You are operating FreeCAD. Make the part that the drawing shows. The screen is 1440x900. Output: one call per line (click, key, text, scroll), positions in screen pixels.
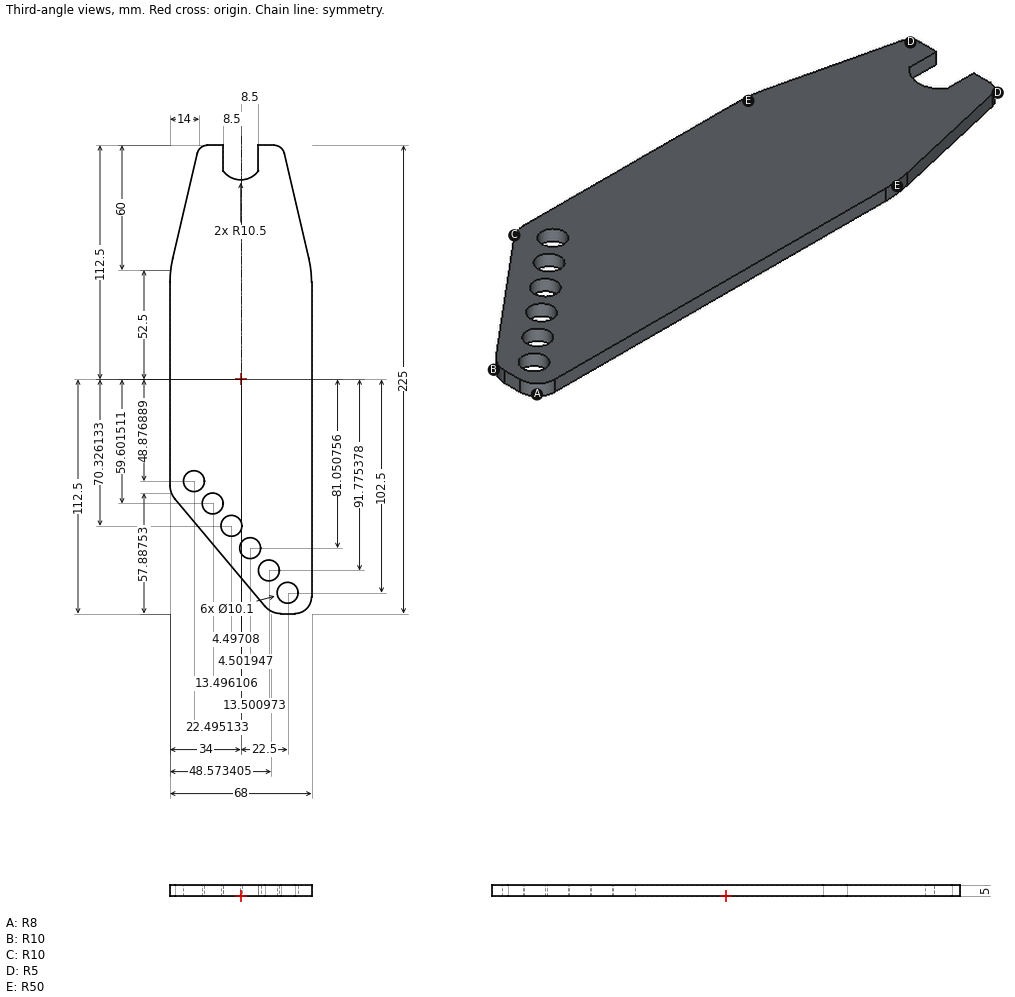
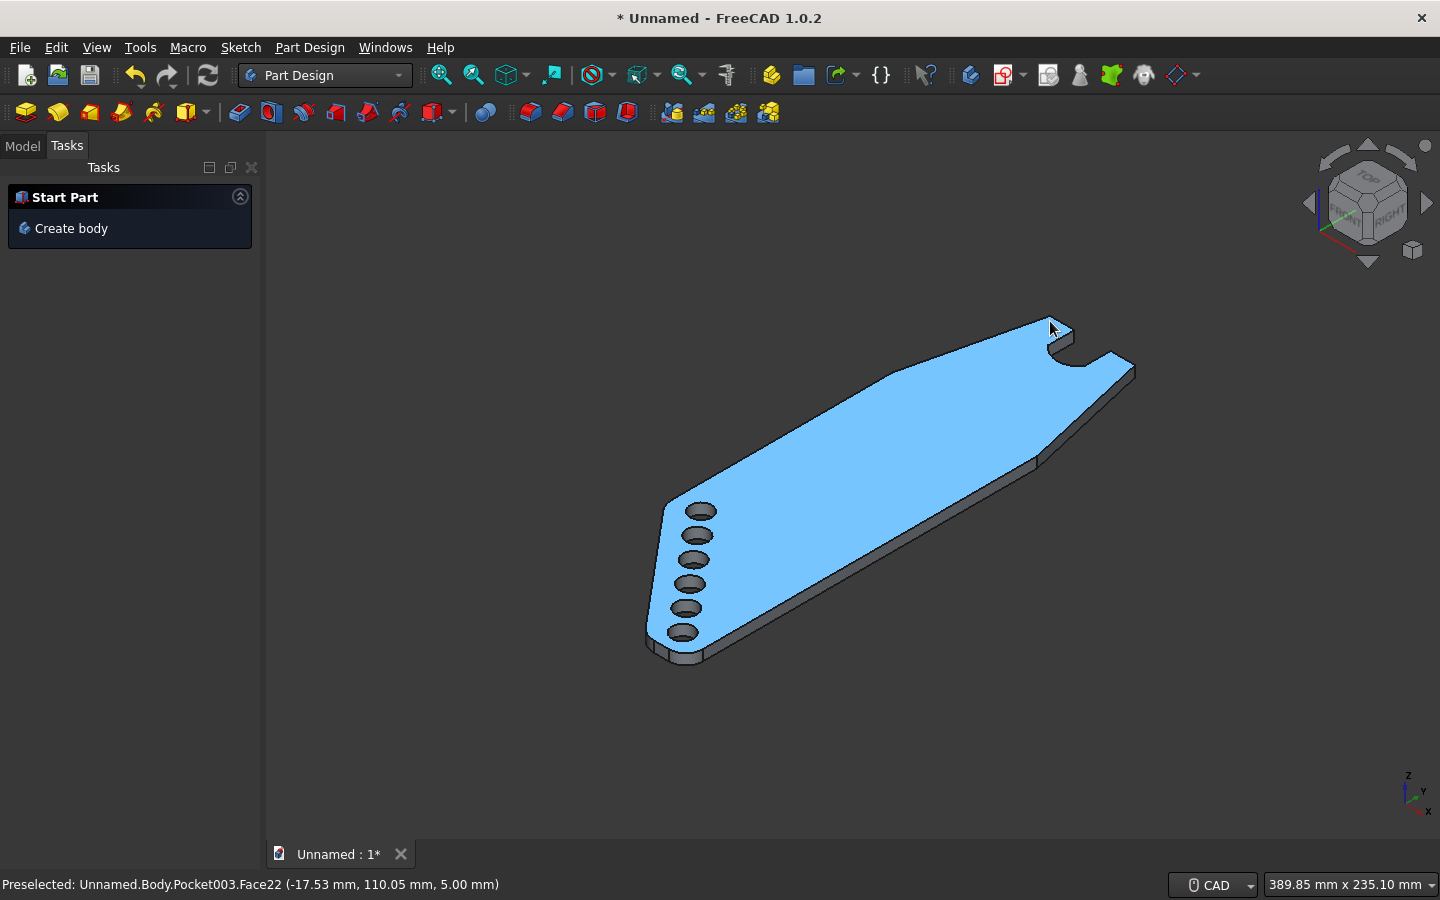
key(2)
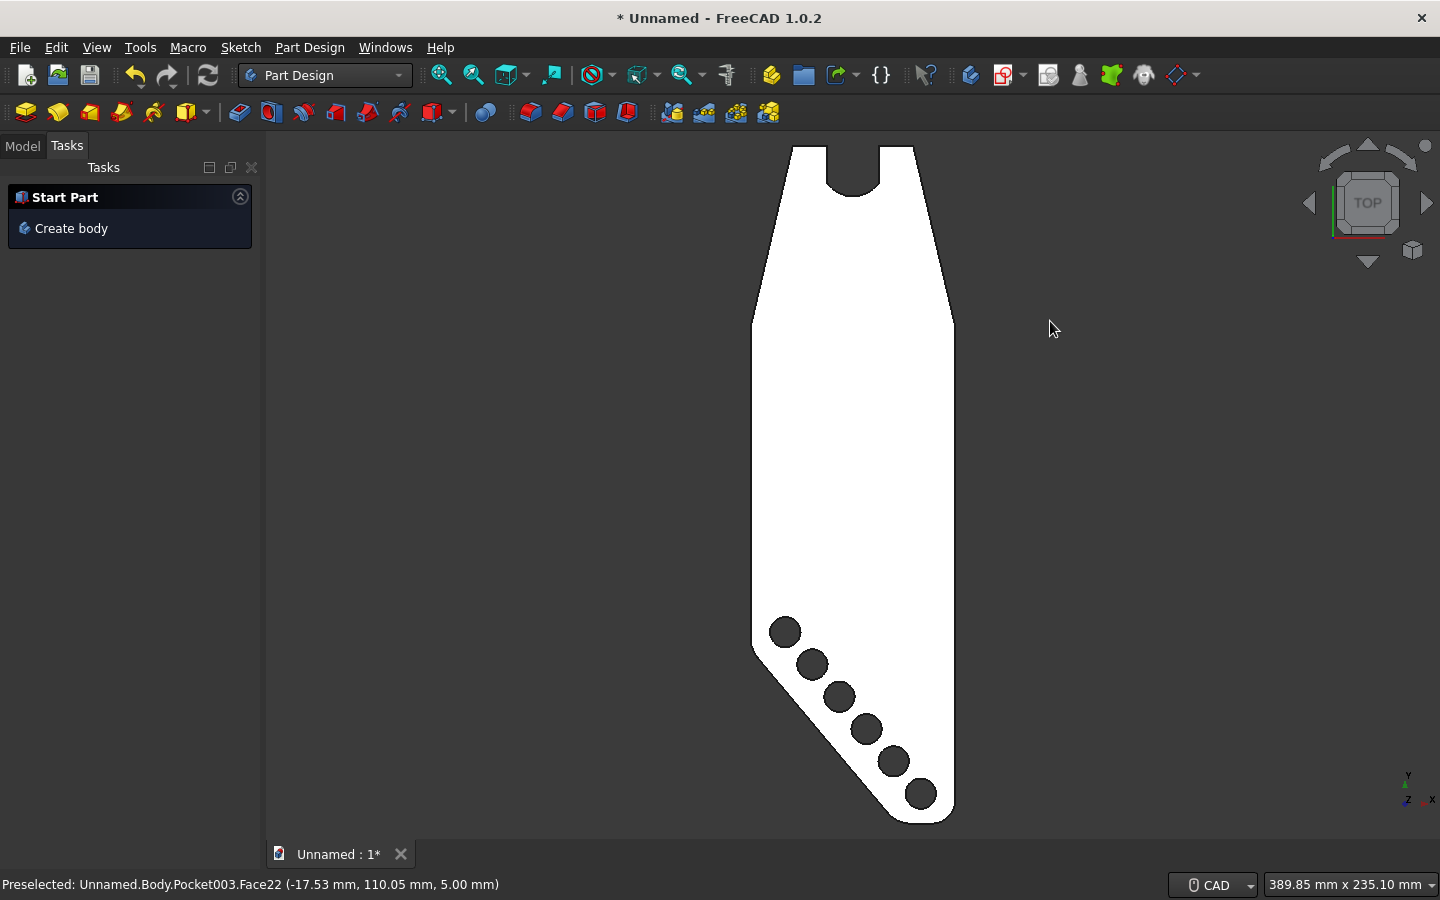
key(0)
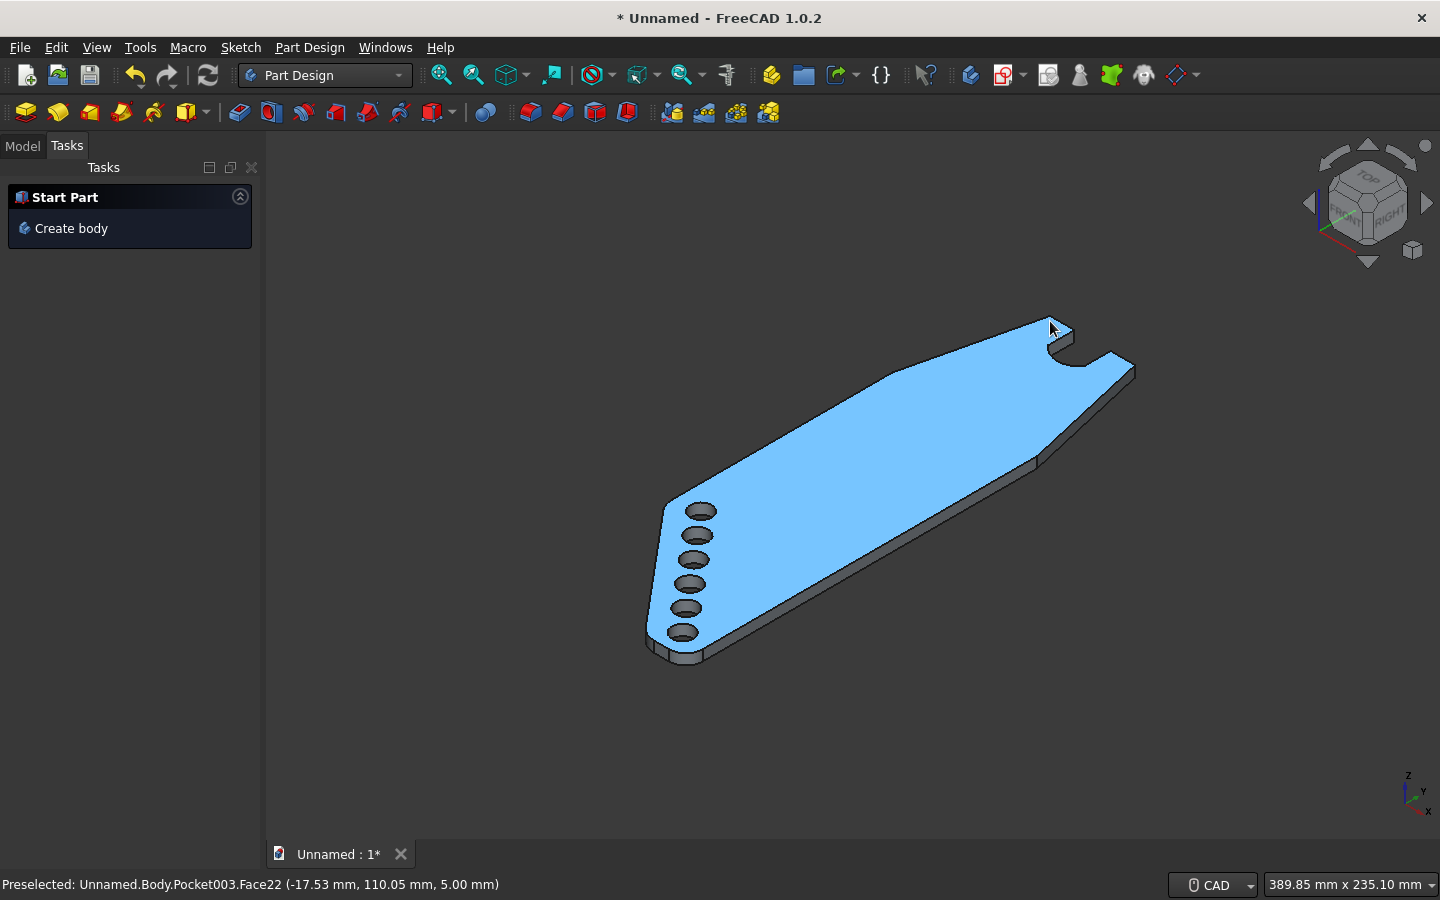
scroll(1050, 321, up, 5)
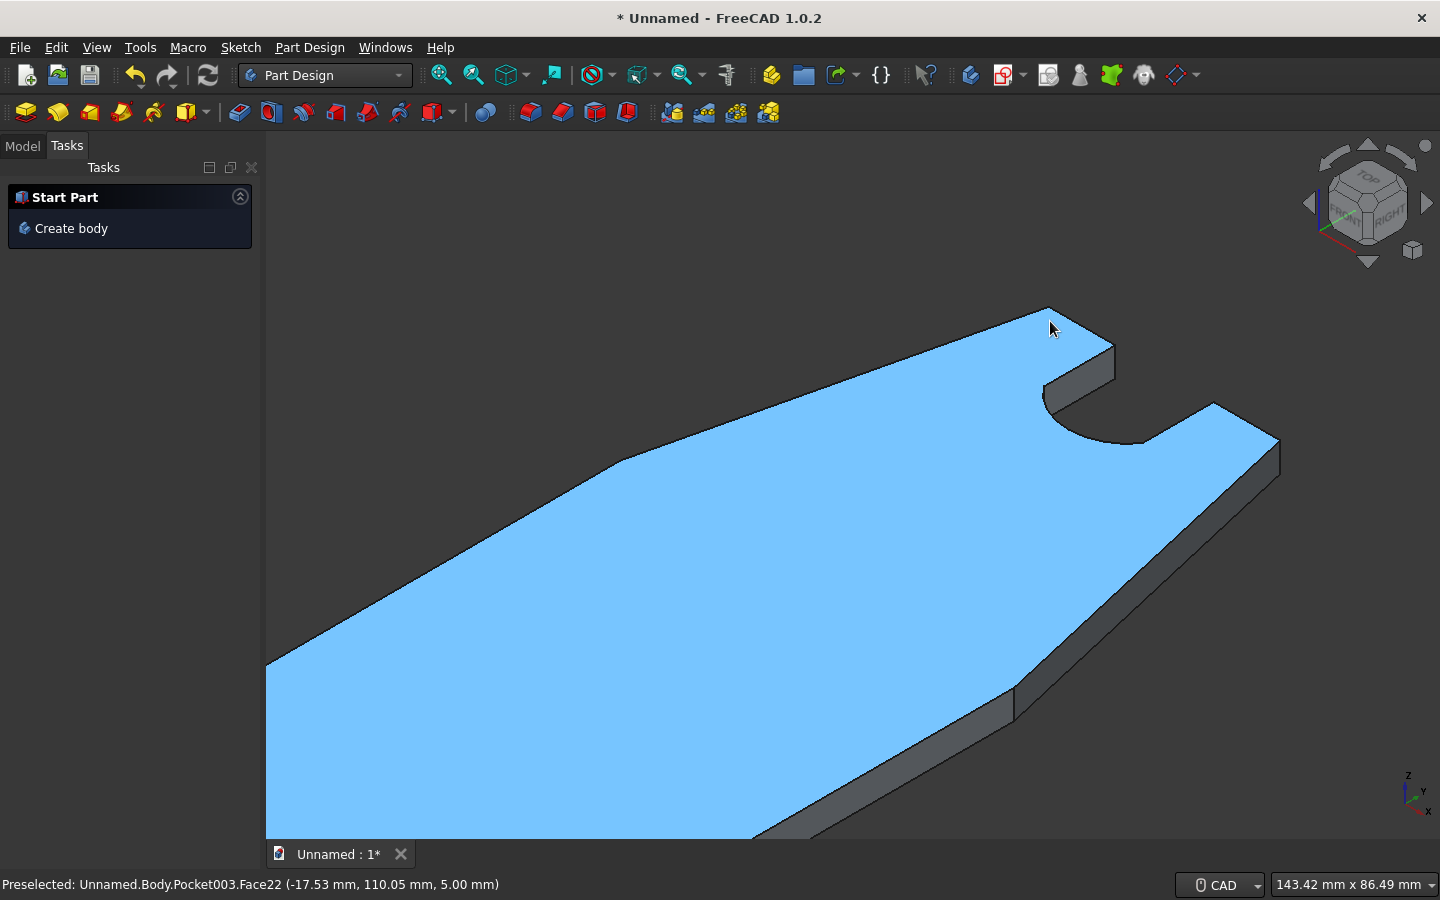
key(v)
key(f)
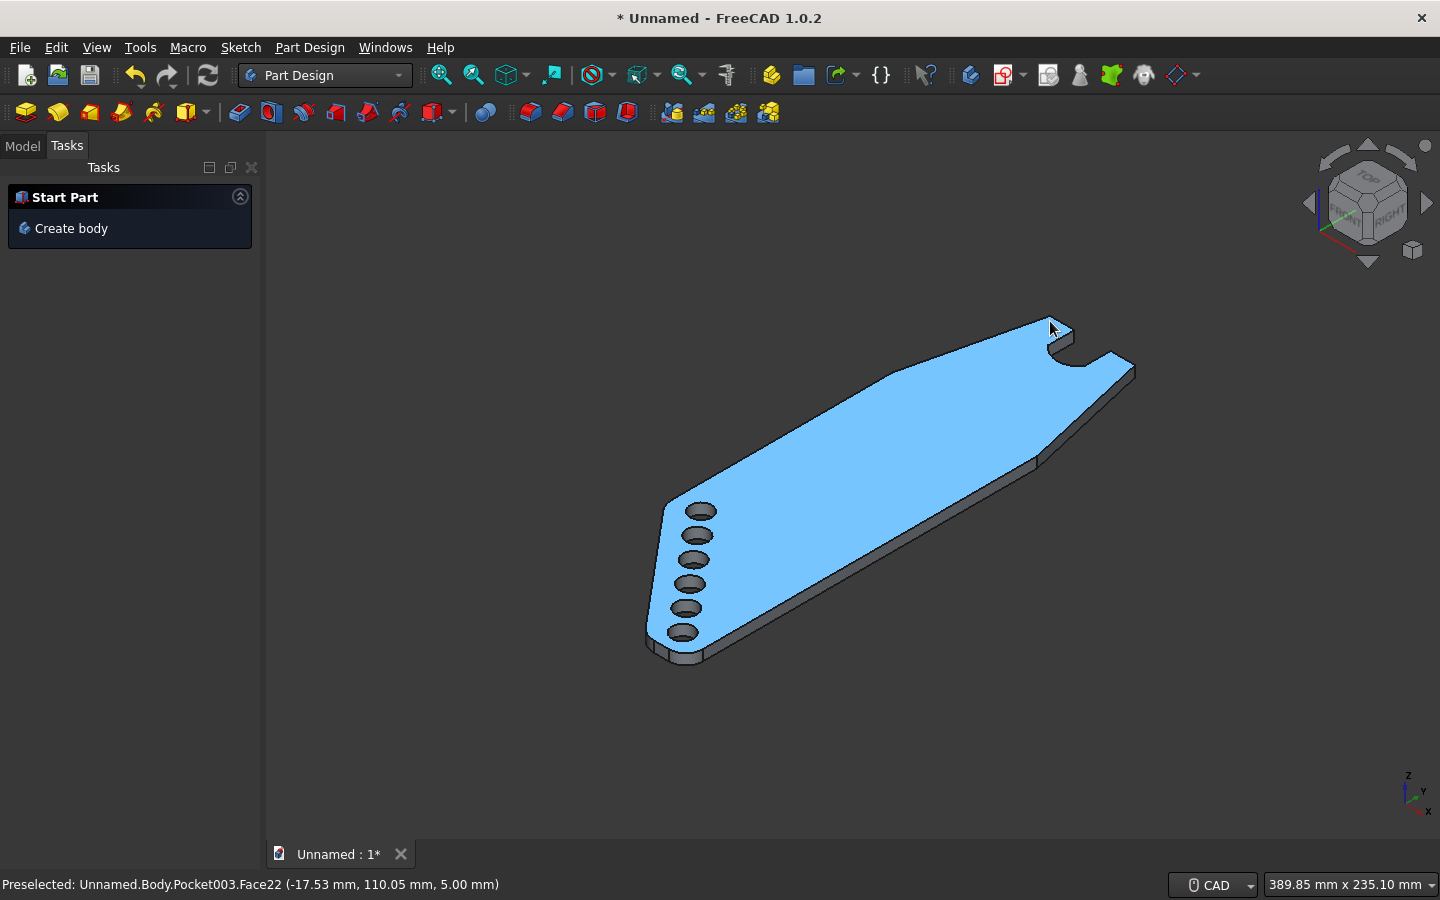
key(1)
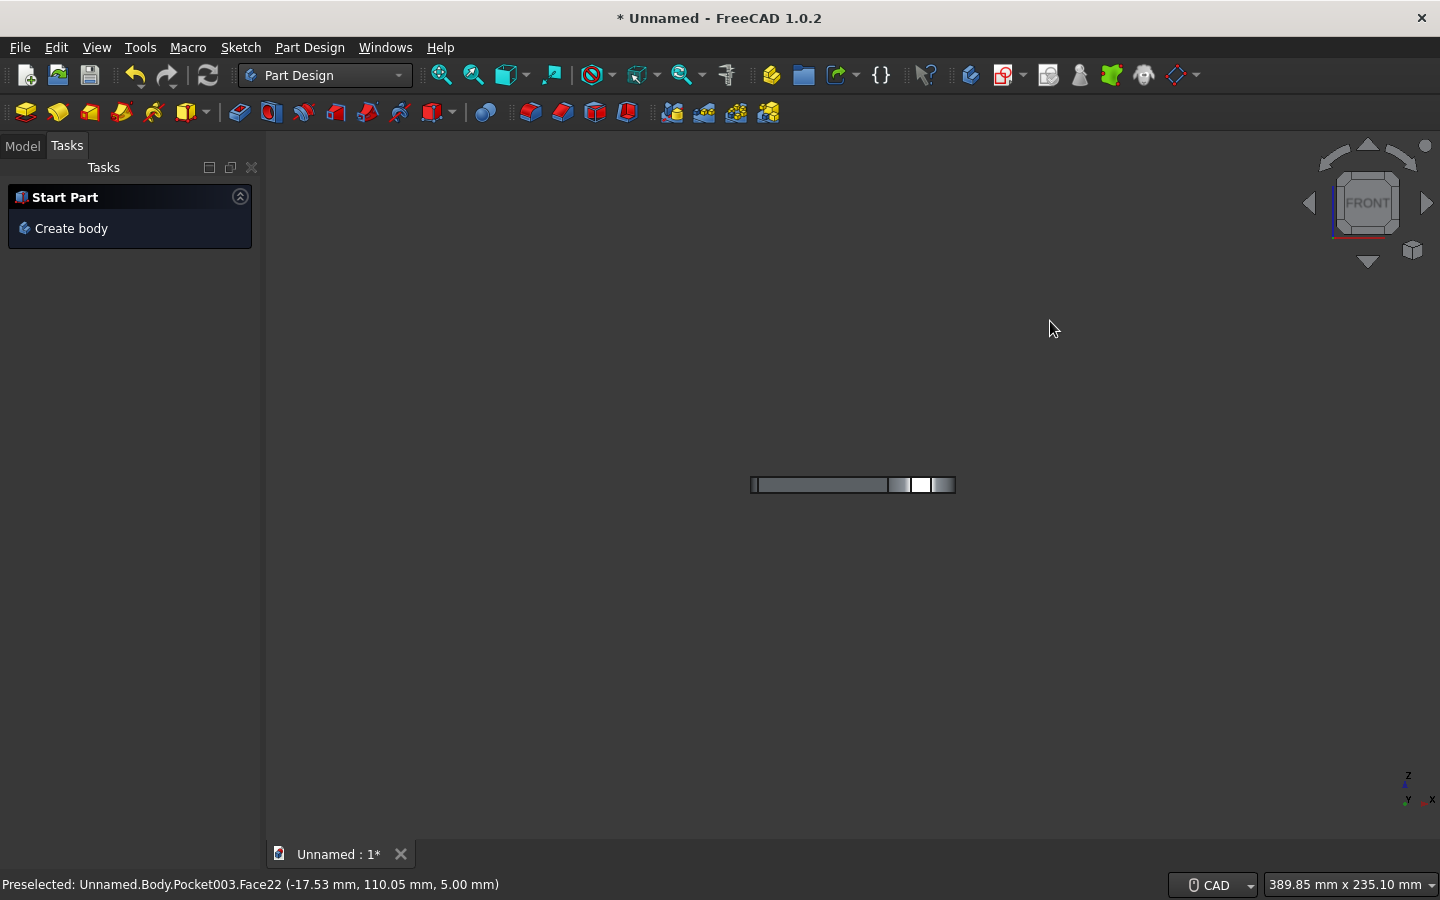
click(442, 76)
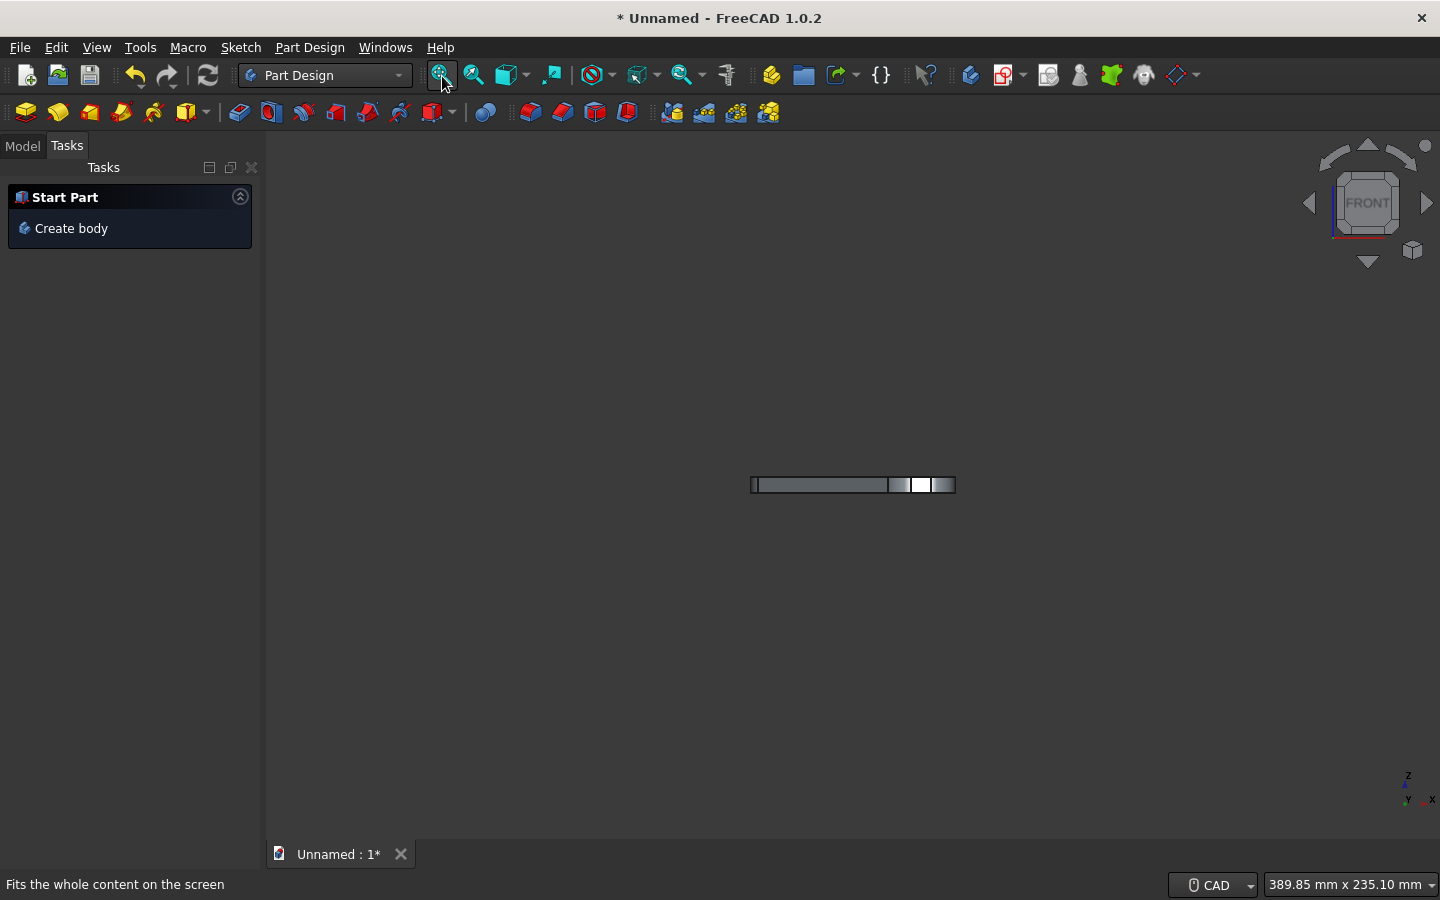
scroll(793, 484, up, 5)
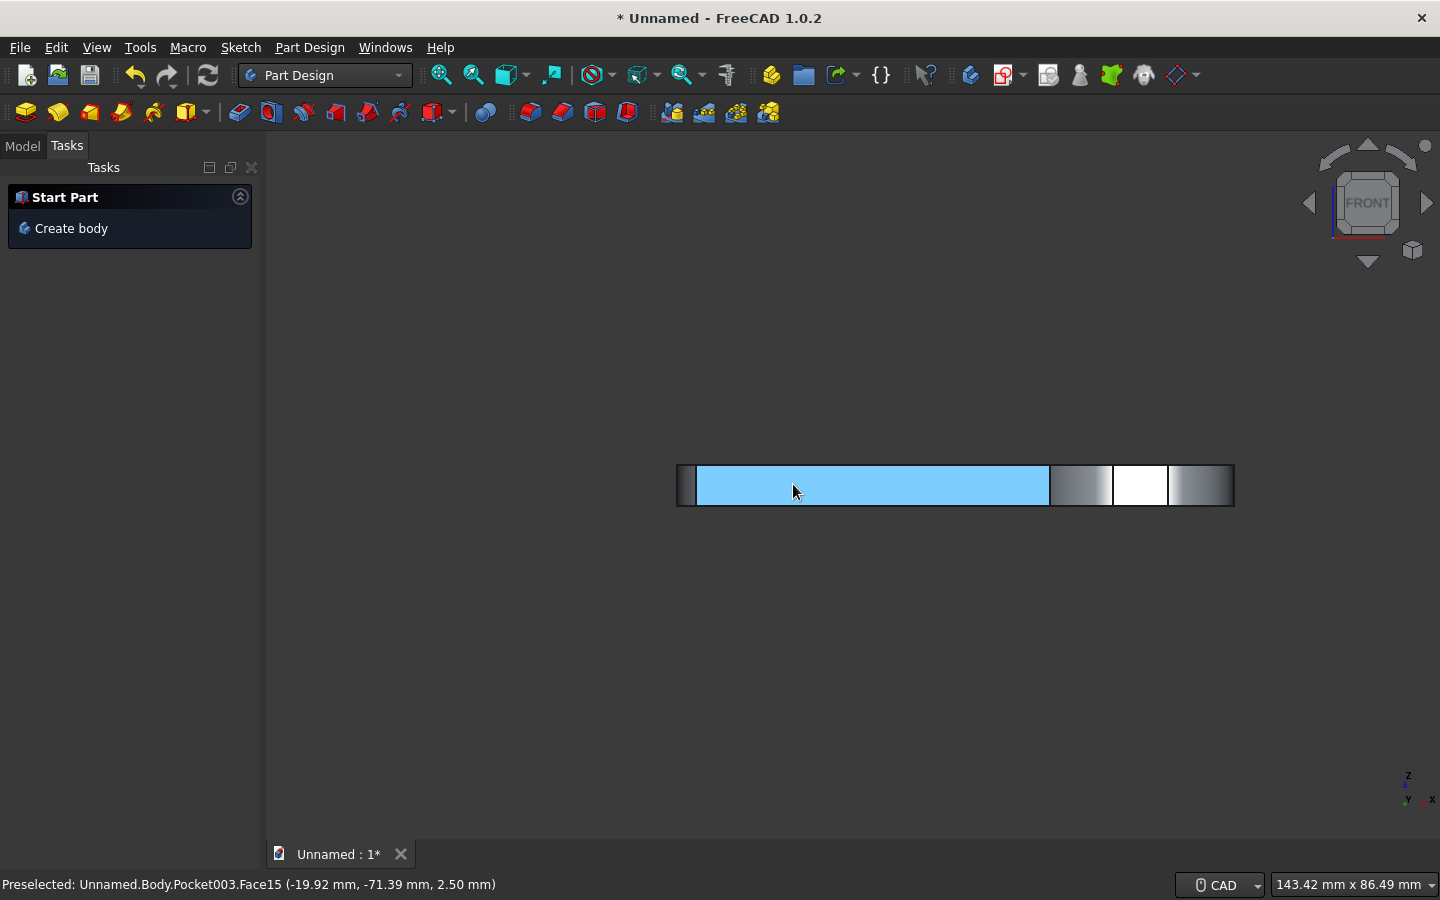
click(442, 76)